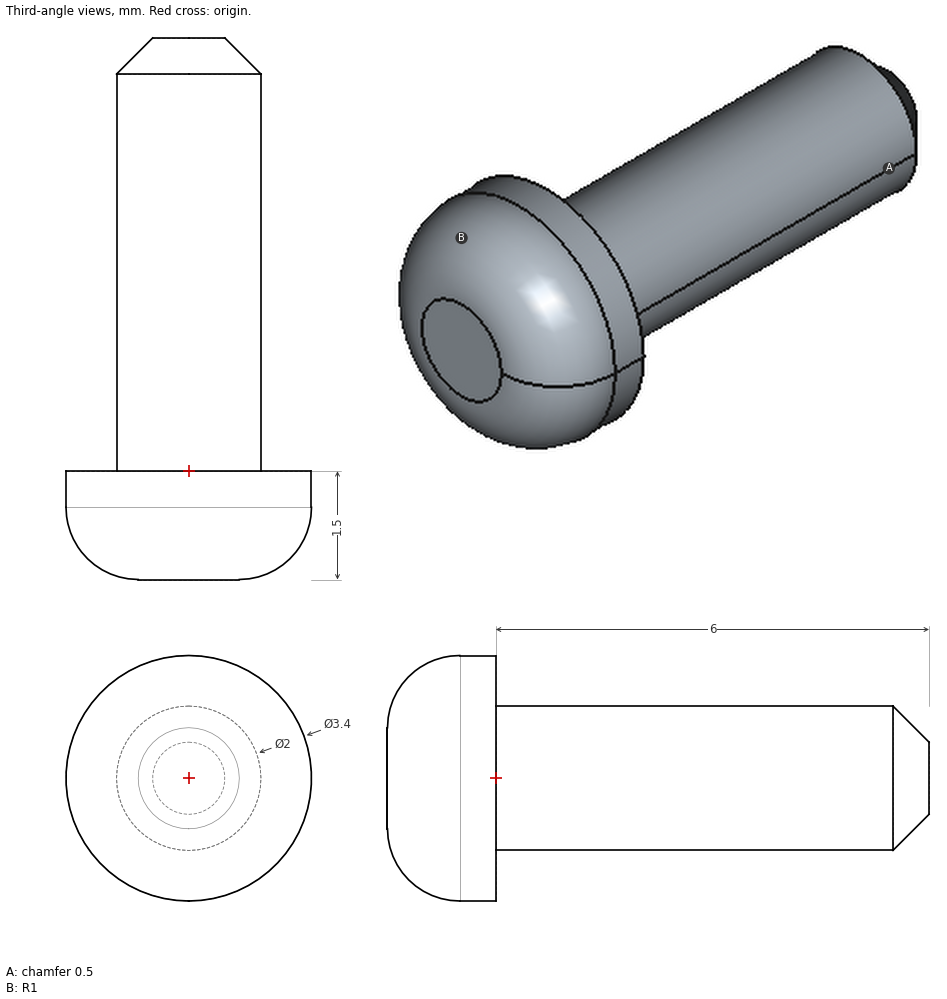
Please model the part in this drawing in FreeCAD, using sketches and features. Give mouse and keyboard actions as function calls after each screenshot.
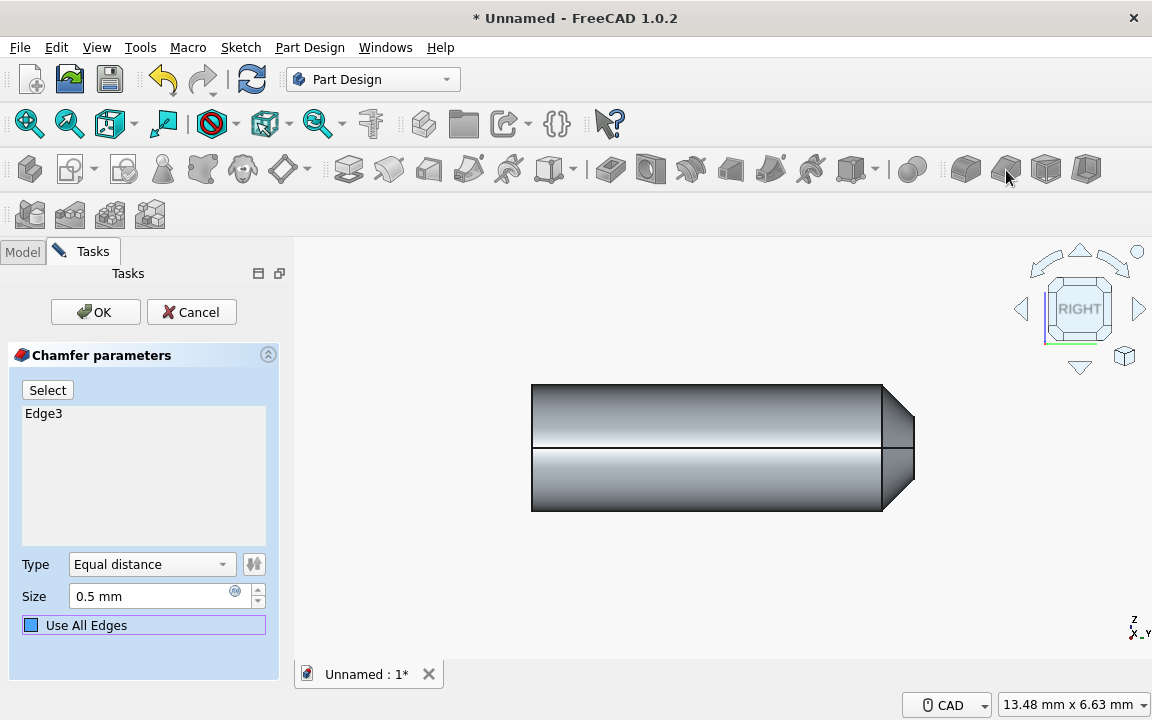
click(96, 312)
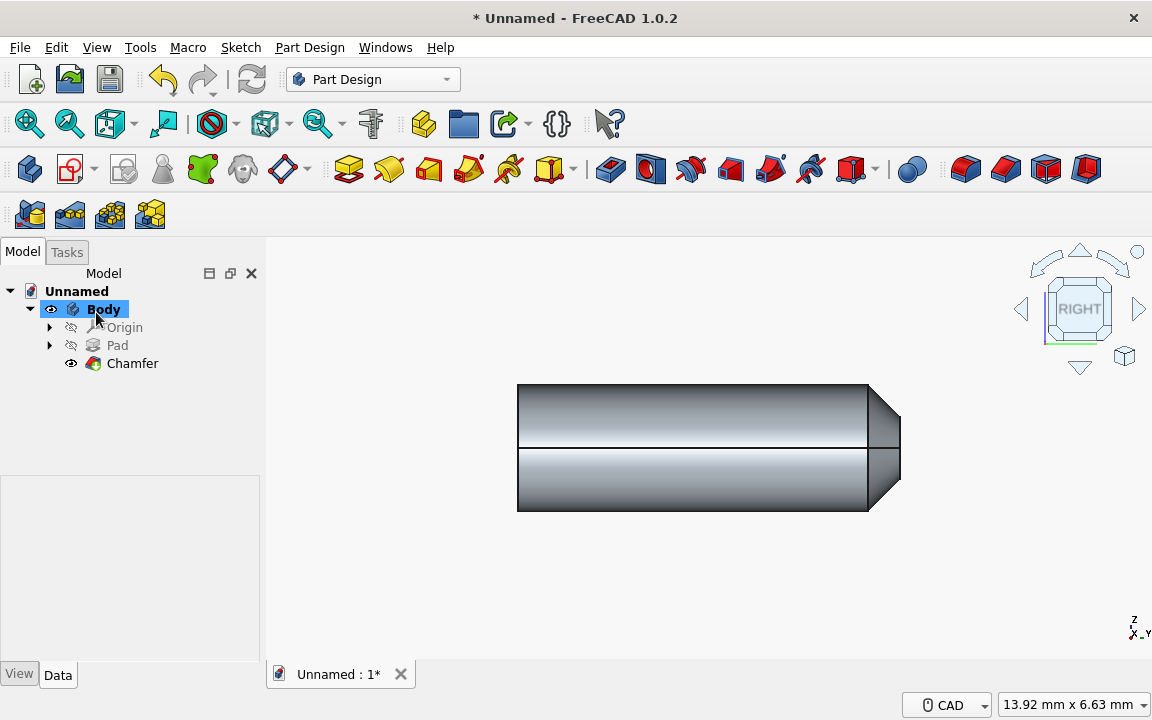
key(v)
key(f)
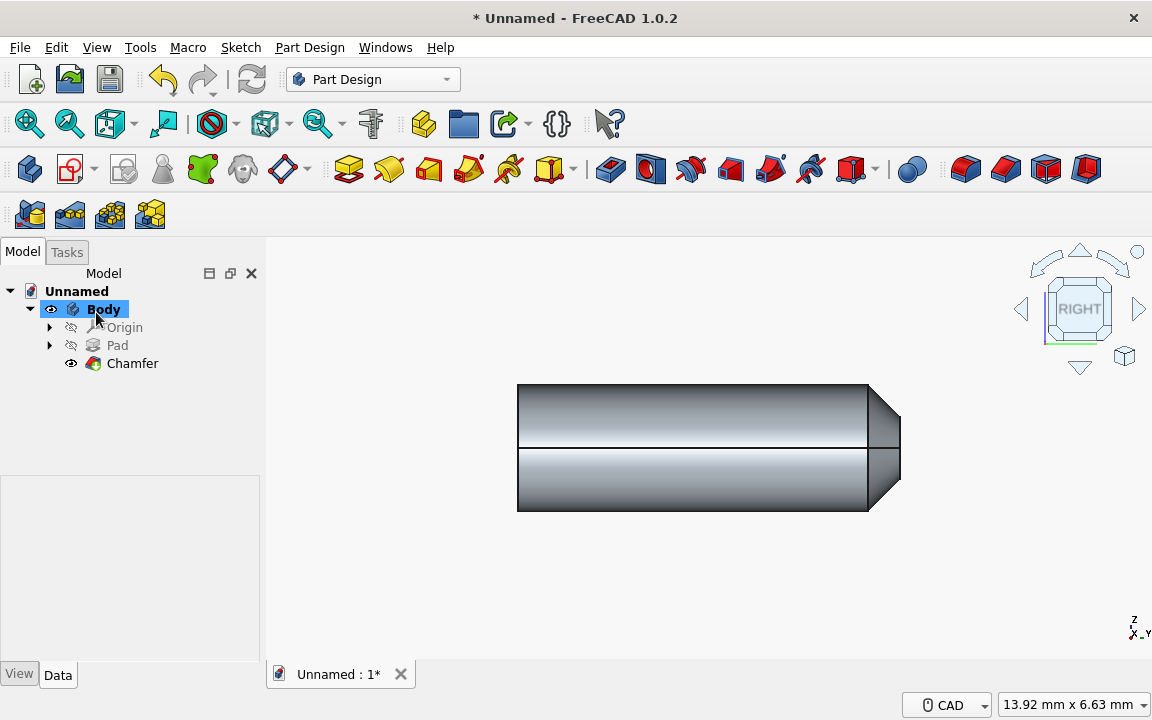
key(0)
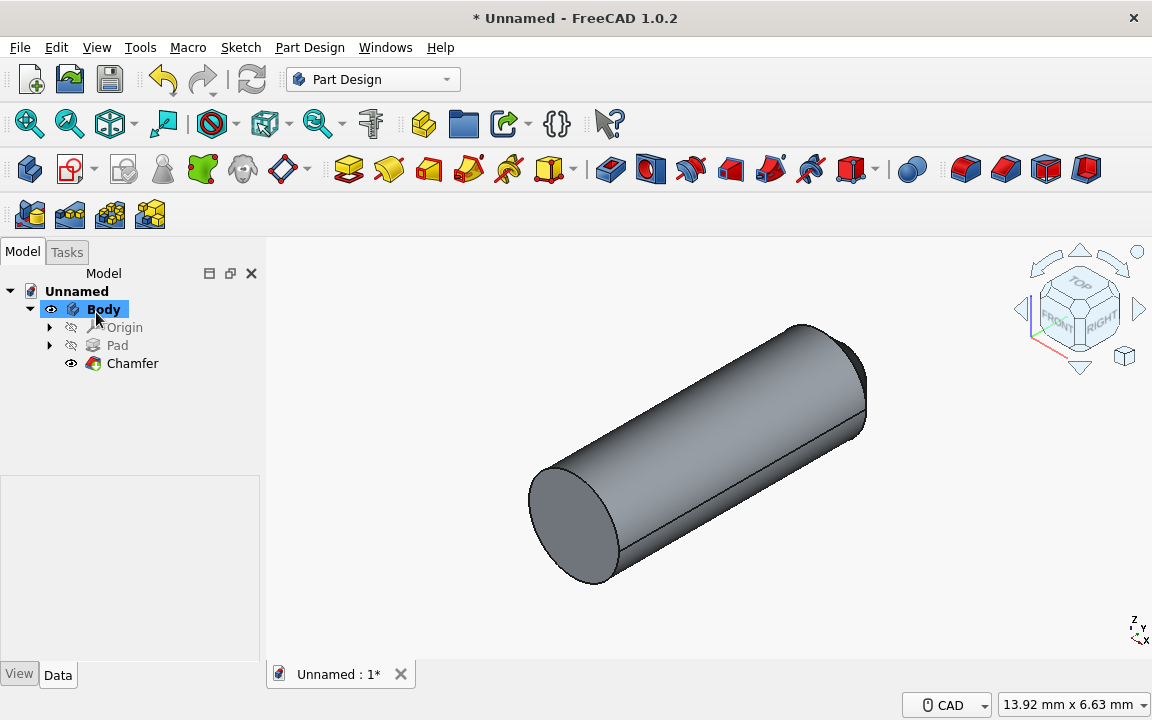
click(574, 525)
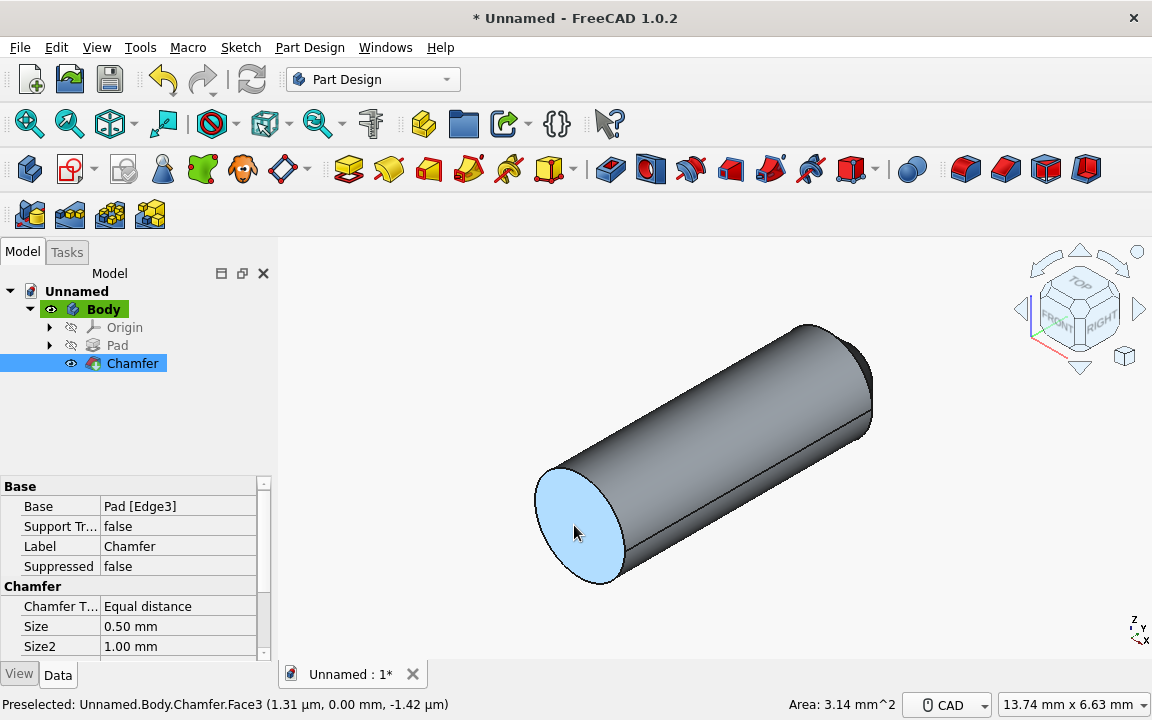
click(70, 170)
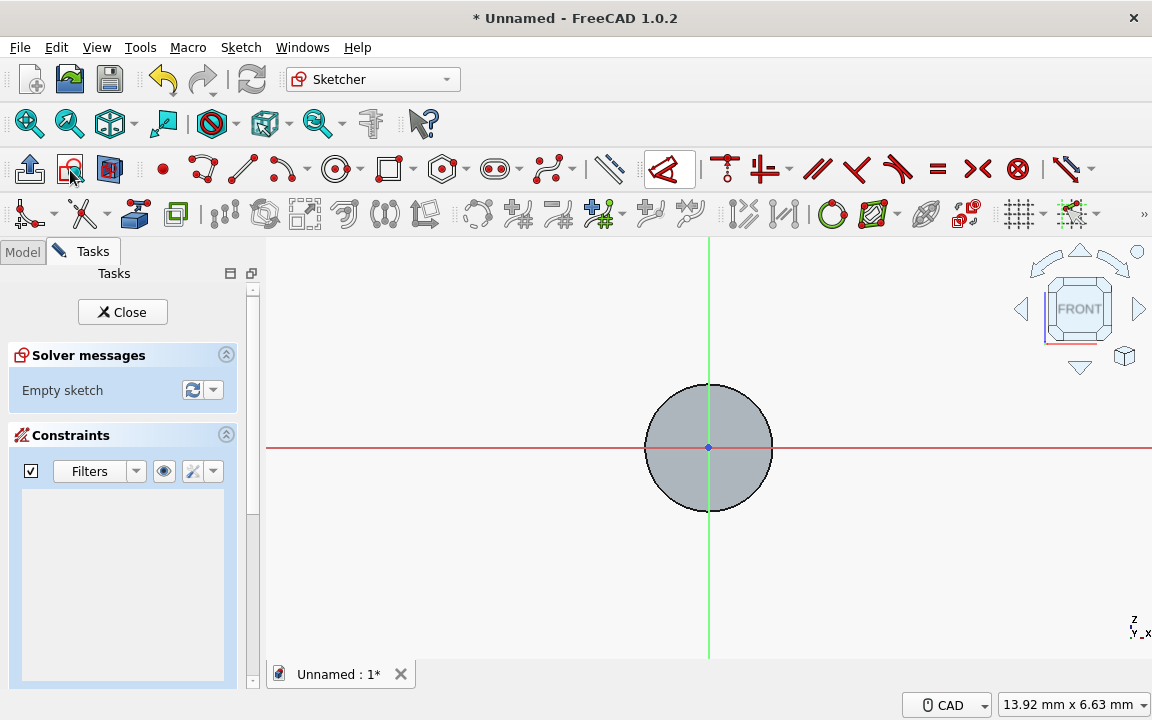
click(336, 170)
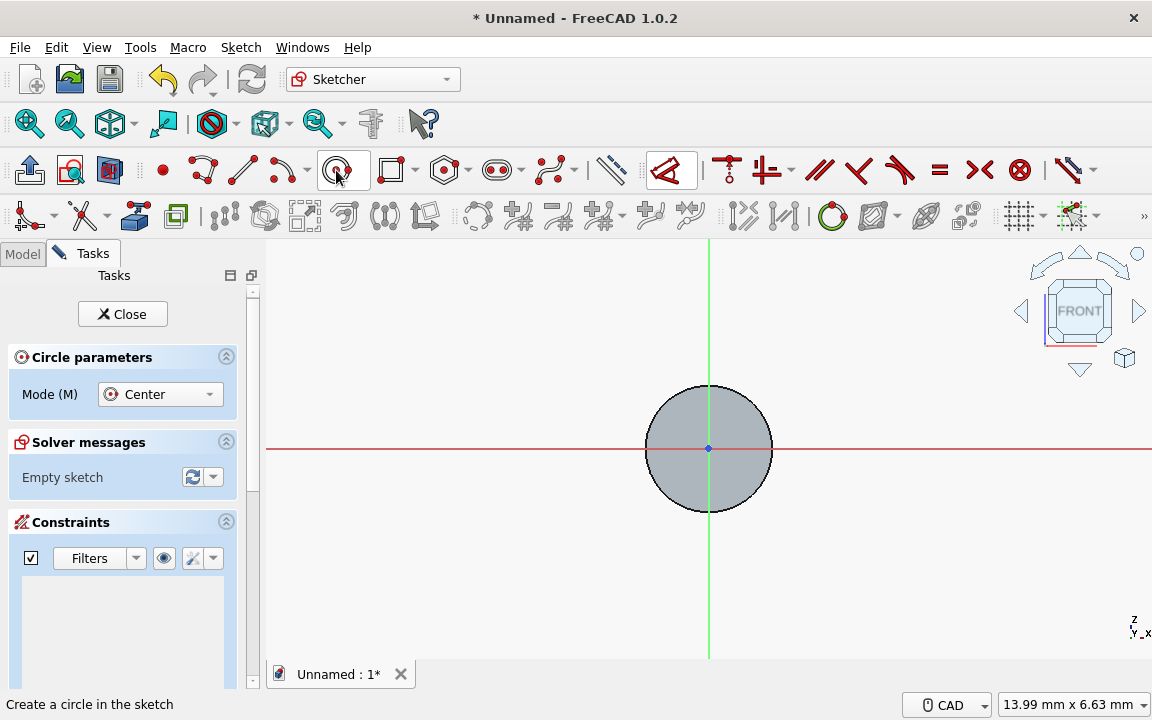
click(709, 449)
move(785, 373)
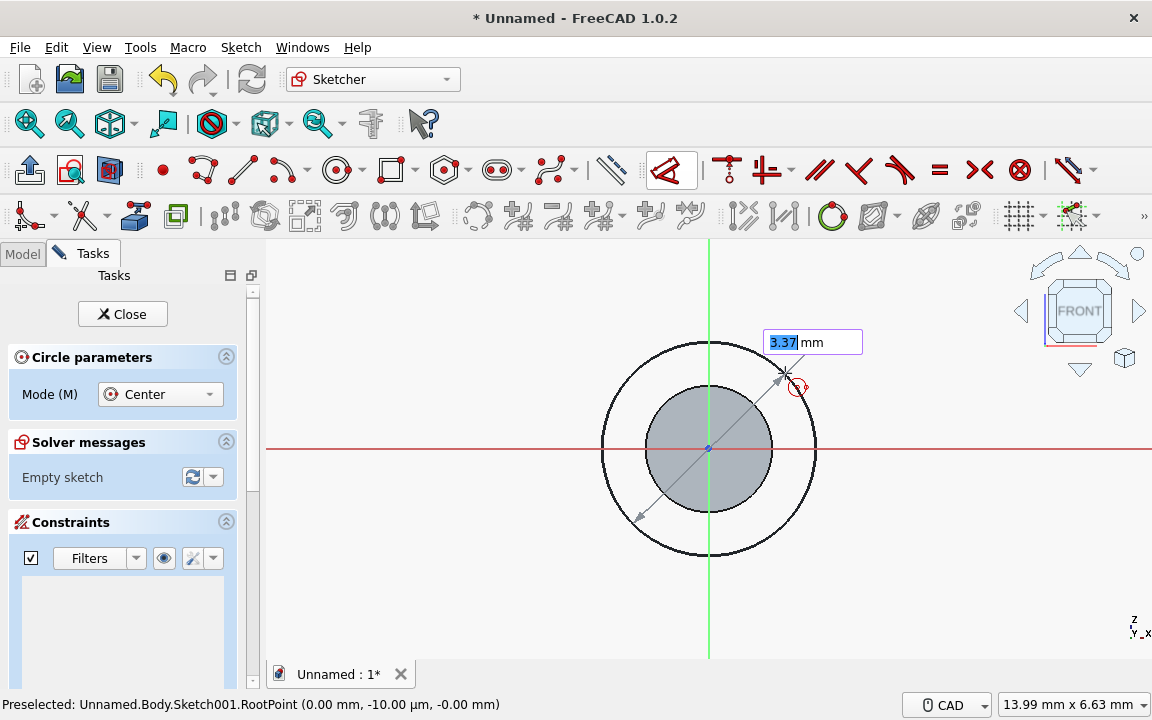
text(3.4)
key(Return)
key(Escape)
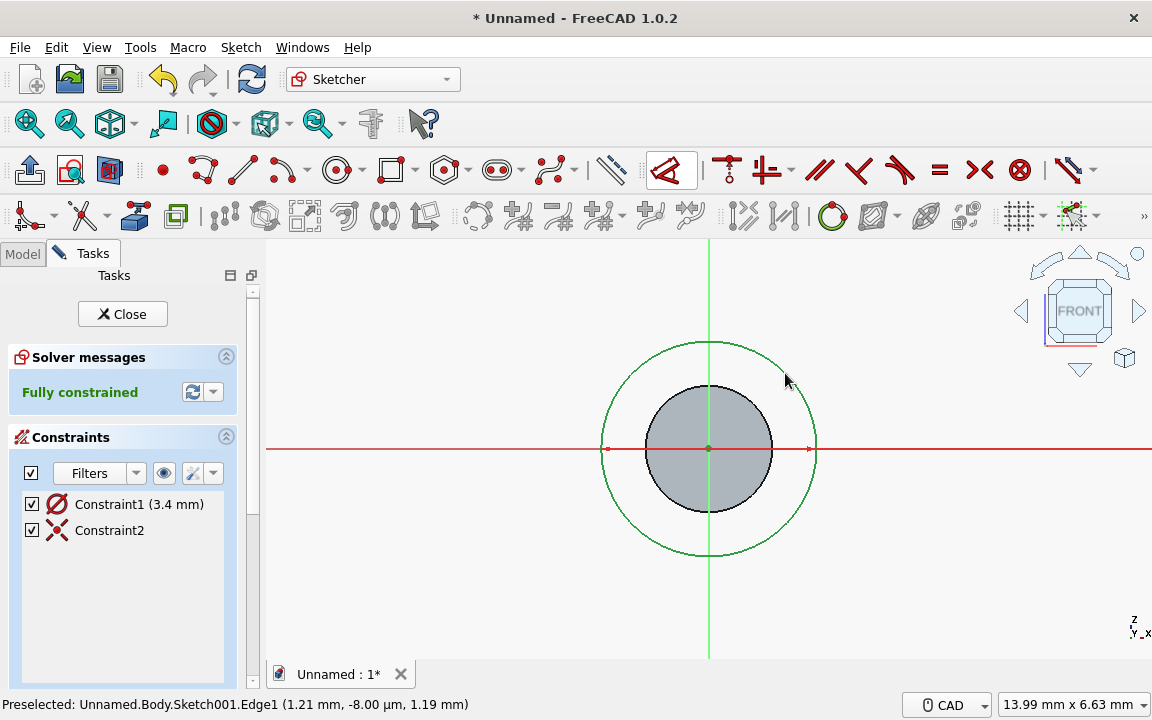
click(123, 314)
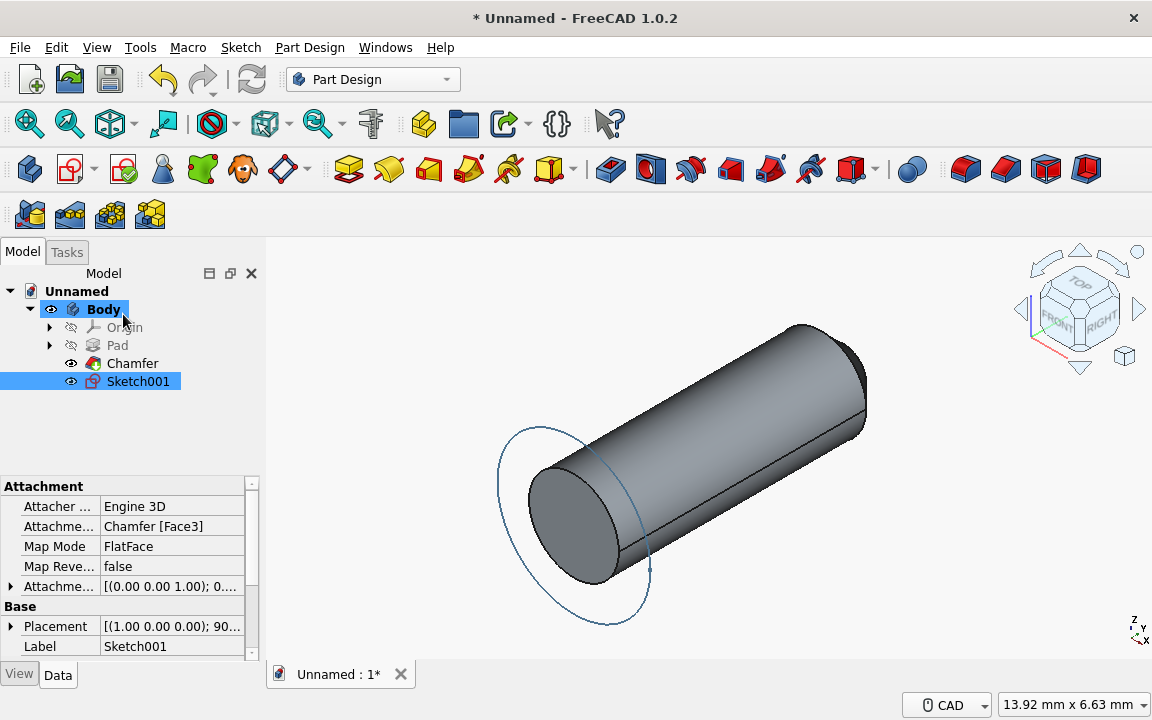
click(350, 170)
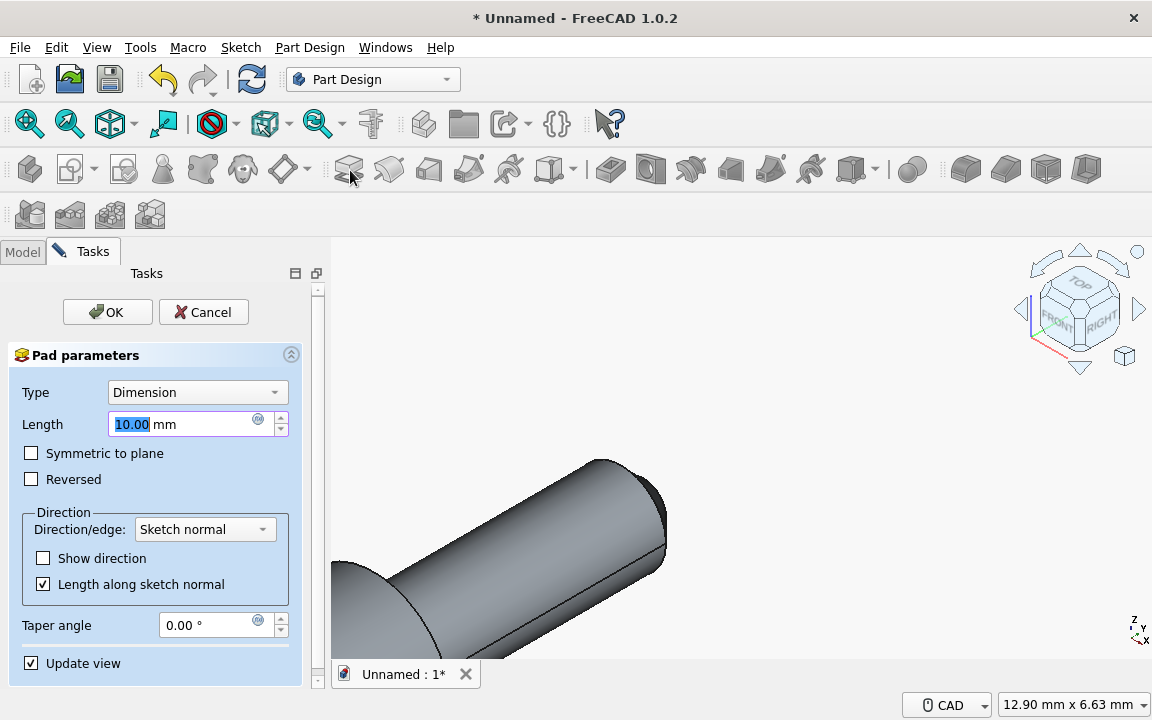
text(1.5)
key(Tab)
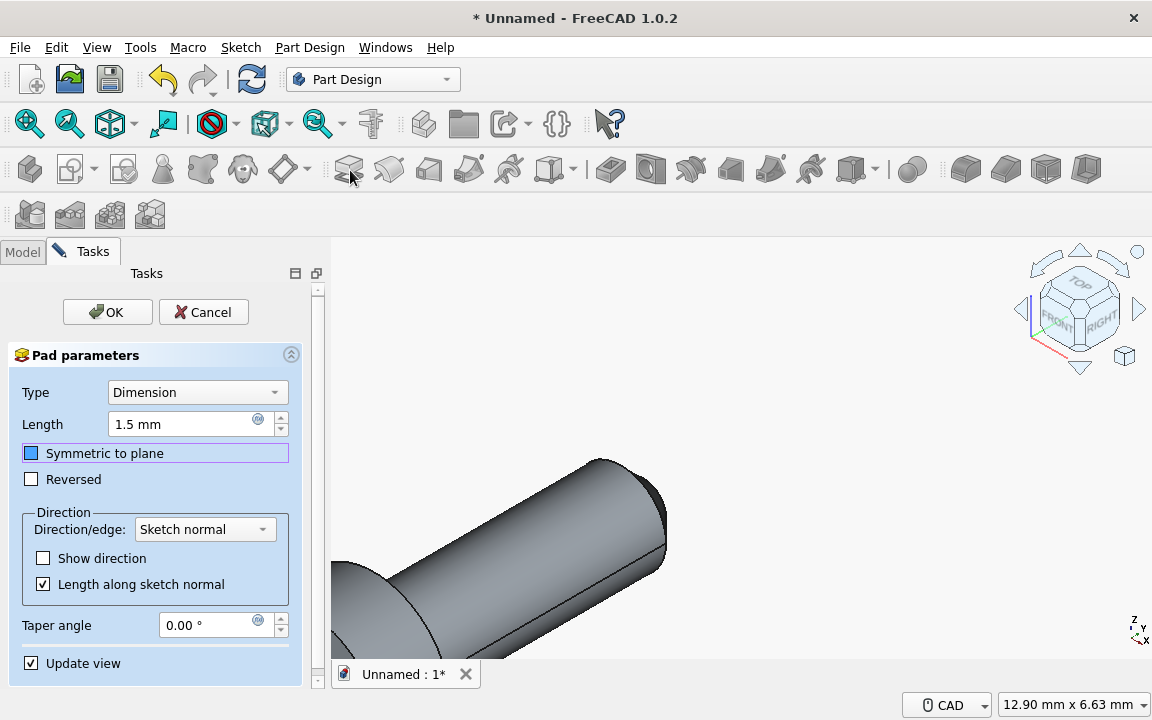
click(108, 312)